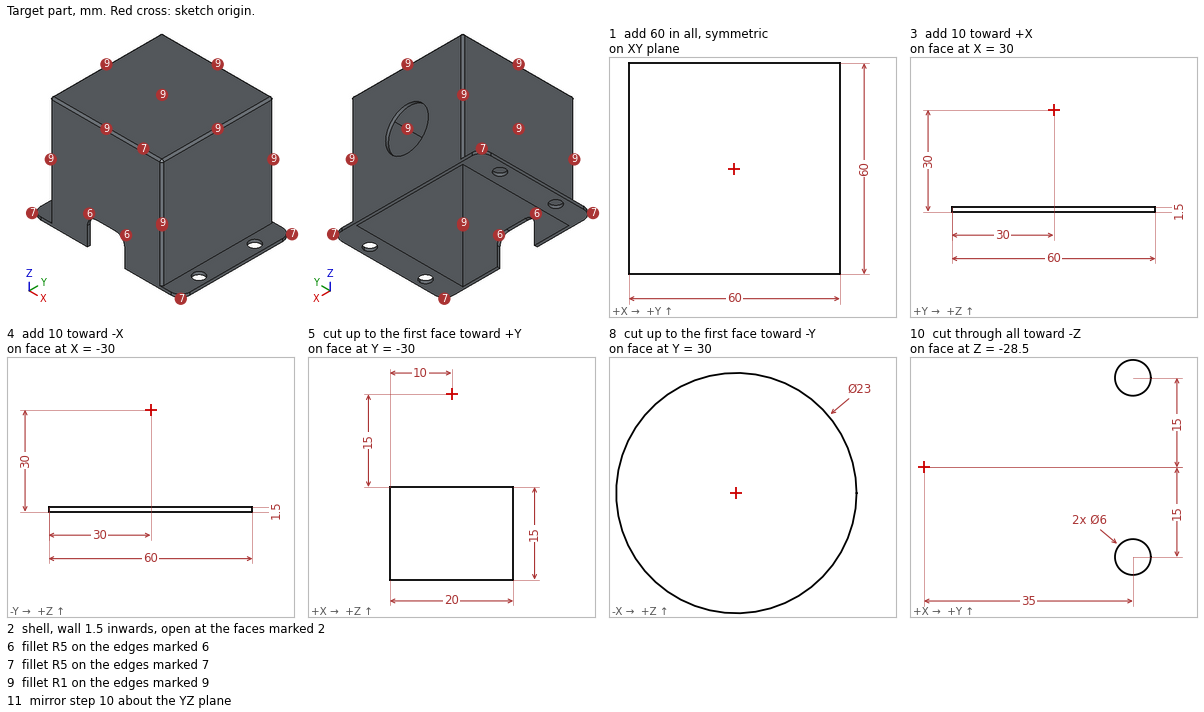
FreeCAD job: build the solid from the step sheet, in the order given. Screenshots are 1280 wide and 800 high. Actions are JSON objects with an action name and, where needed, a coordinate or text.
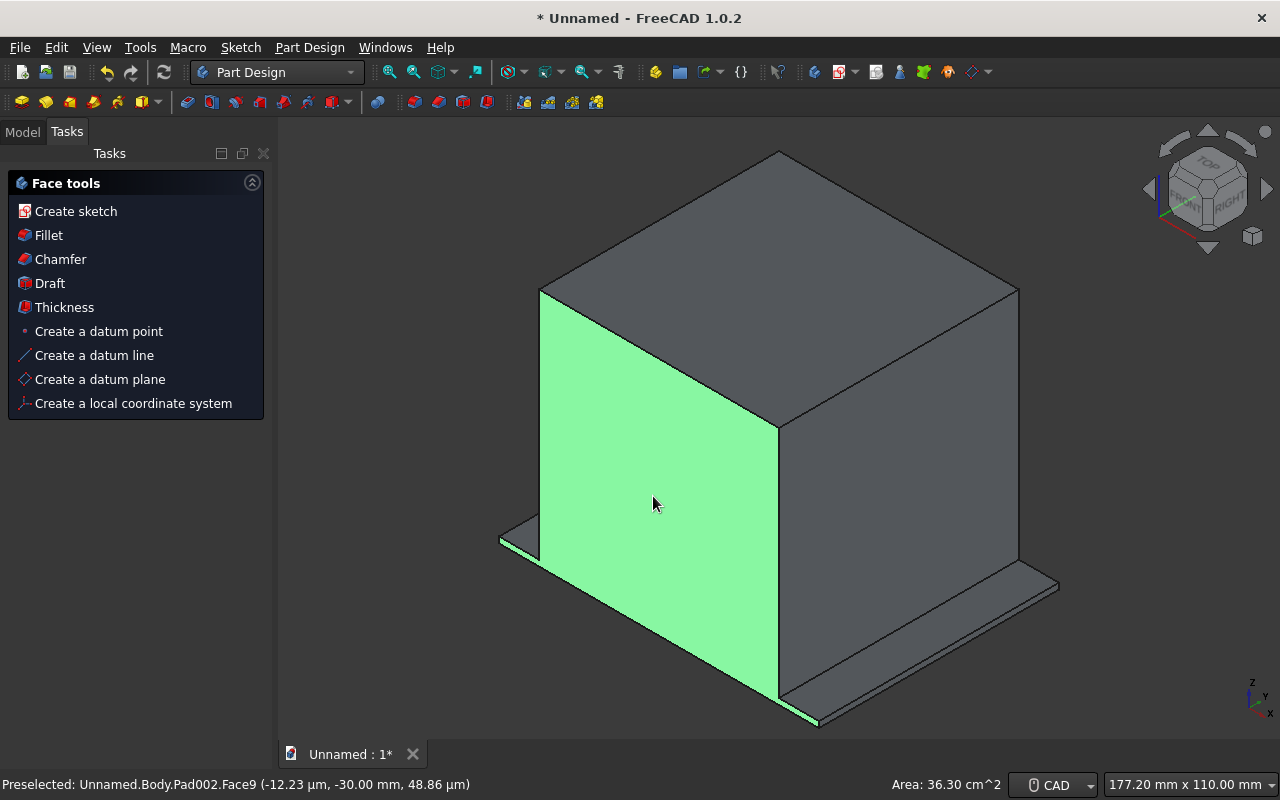
{"action": "left_click", "coordinate": [840, 72]}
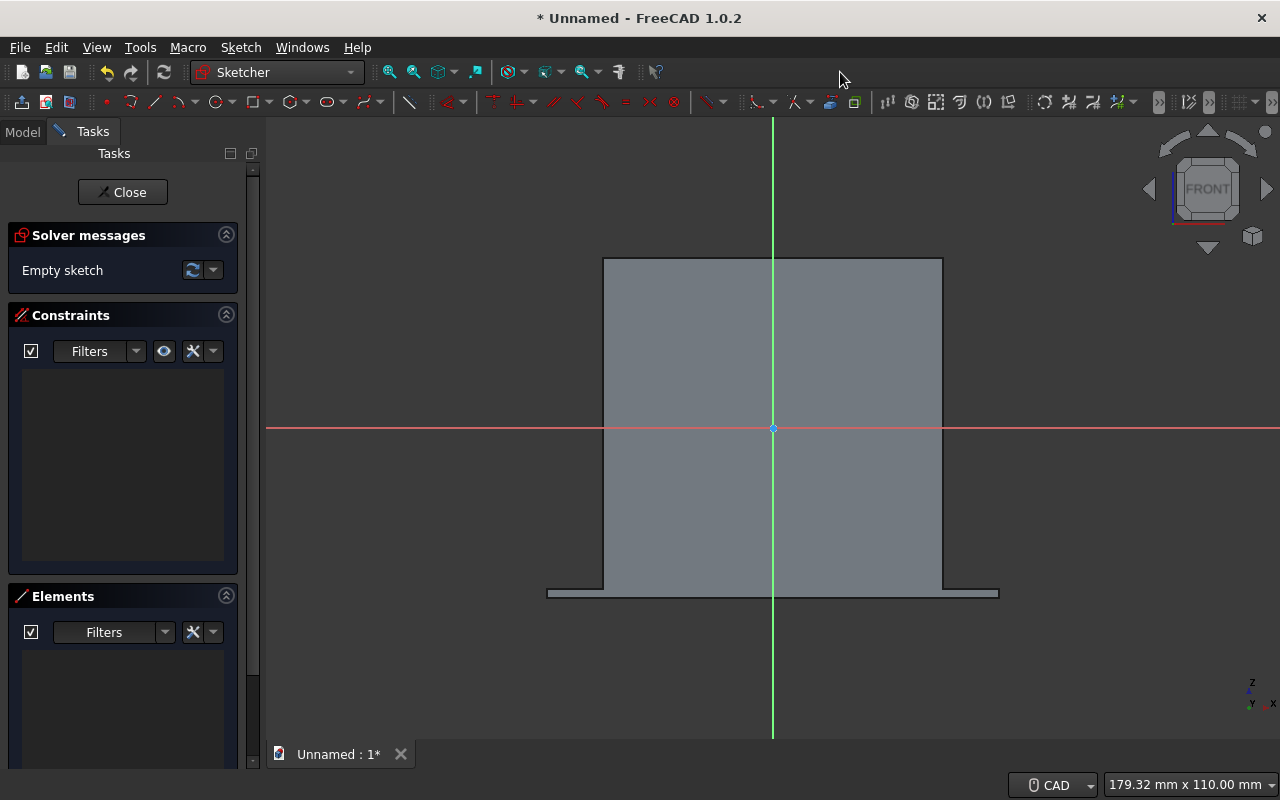
{"action": "scroll", "coordinate": [829, 582], "scroll_direction": "up", "scroll_amount": 4}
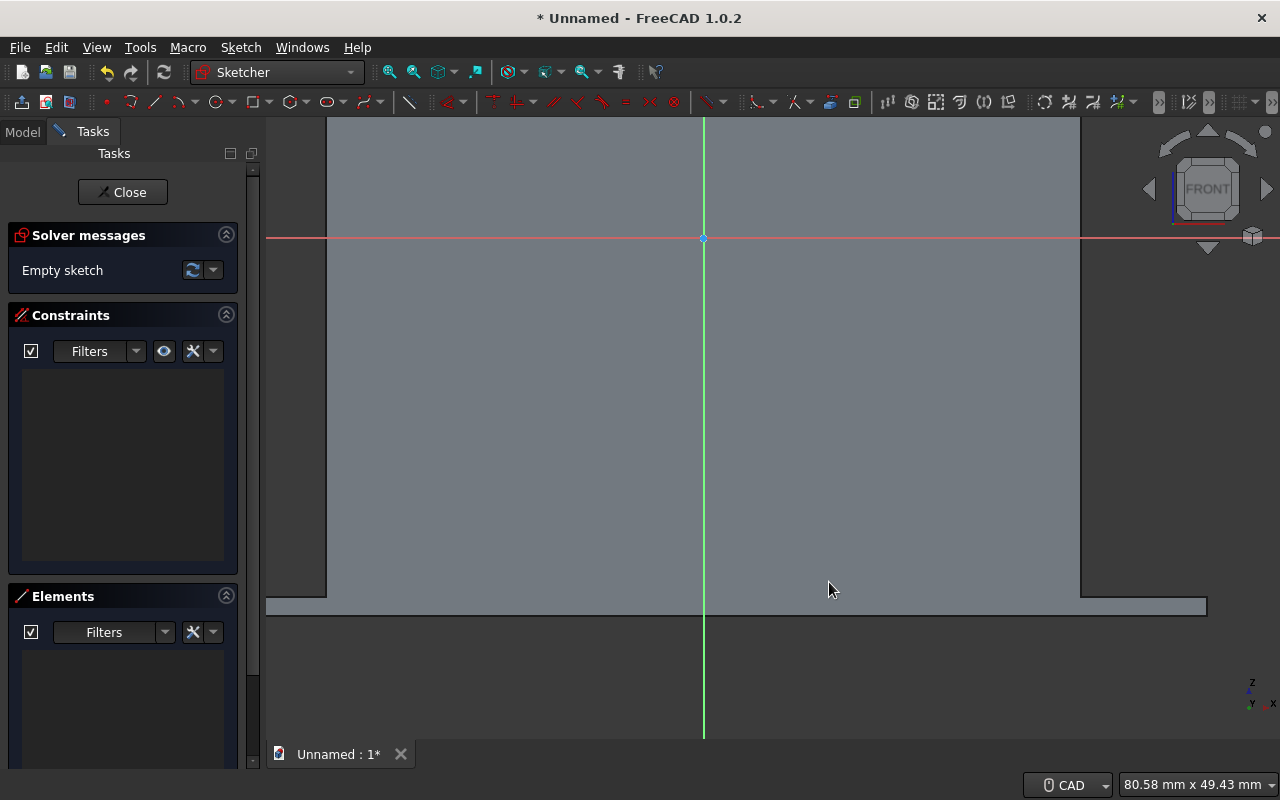
{"action": "left_click", "coordinate": [254, 102]}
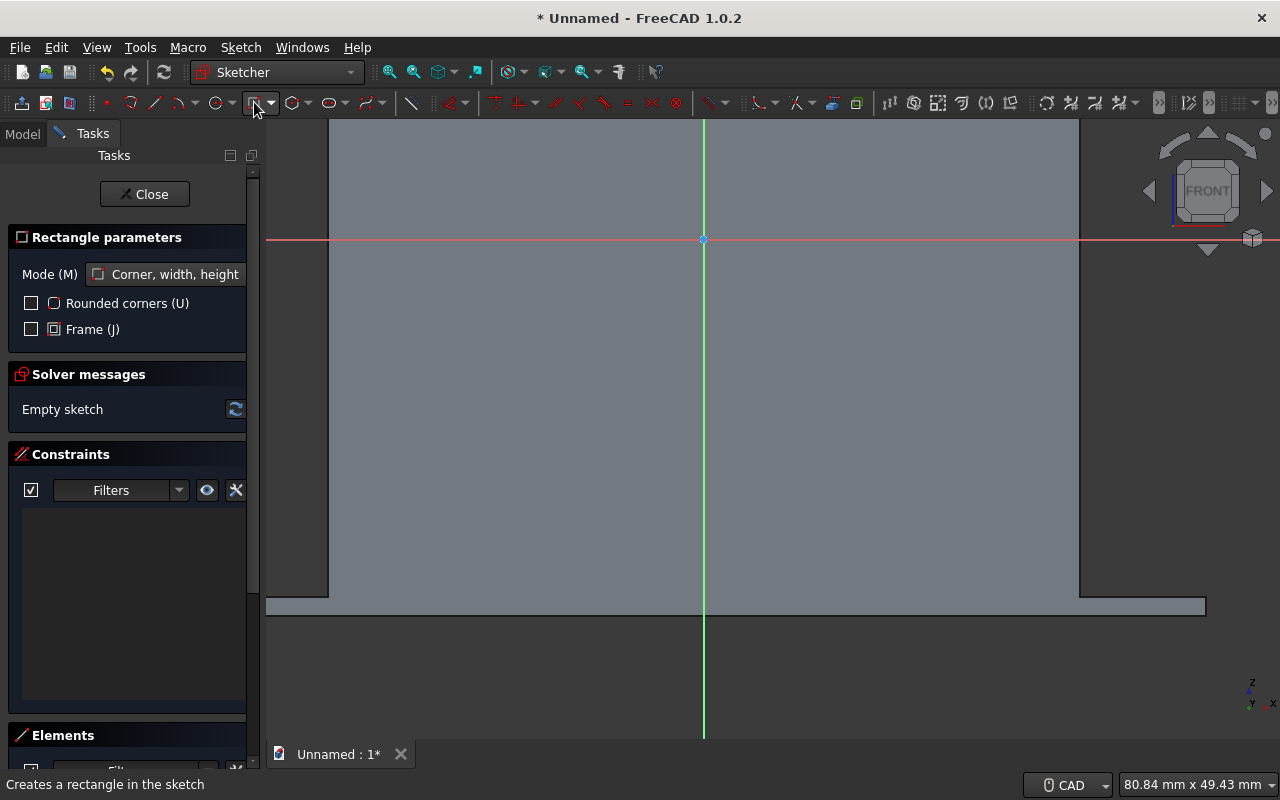
{"action": "left_click", "coordinate": [578, 428]}
{"action": "mouse_move", "coordinate": [829, 616]}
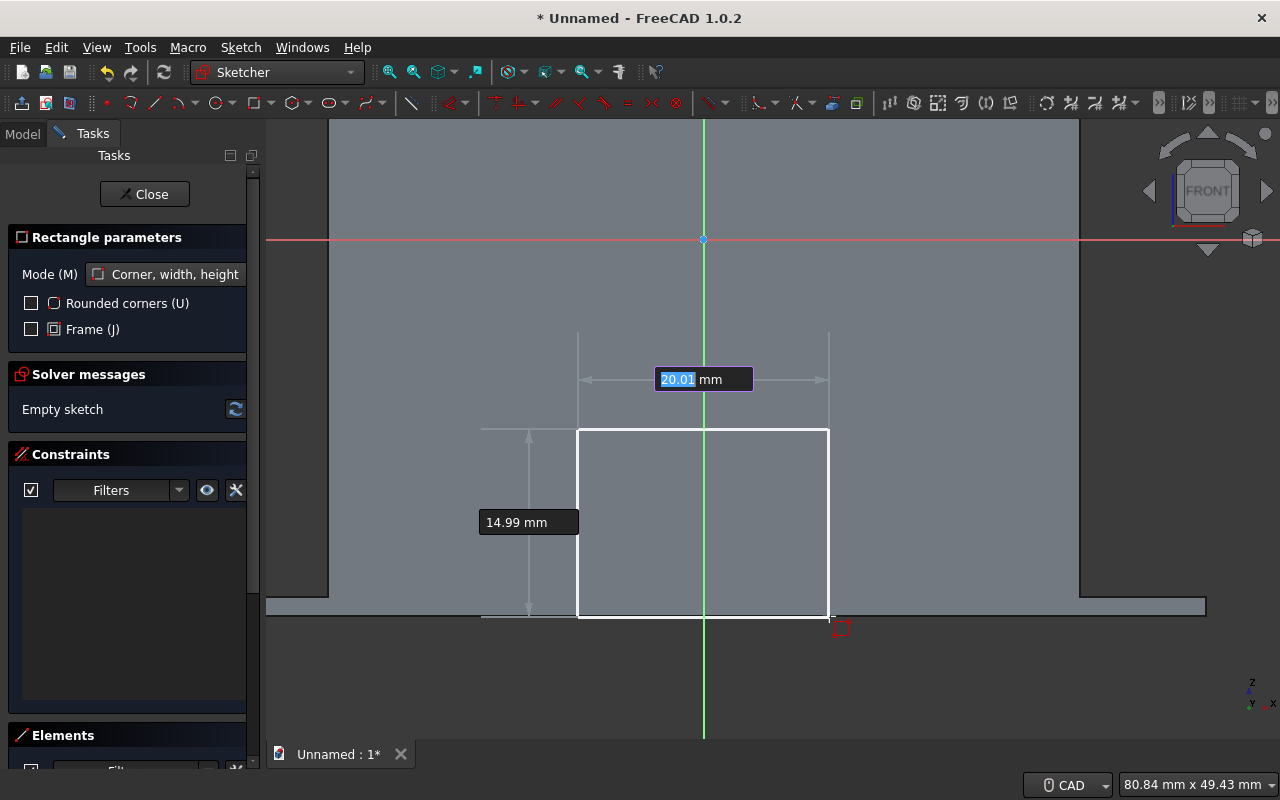
{"action": "type", "text": "20"}
{"action": "key", "text": "Tab"}
{"action": "type", "text": "15"}
{"action": "key", "text": "Return"}
{"action": "key", "text": "Escape"}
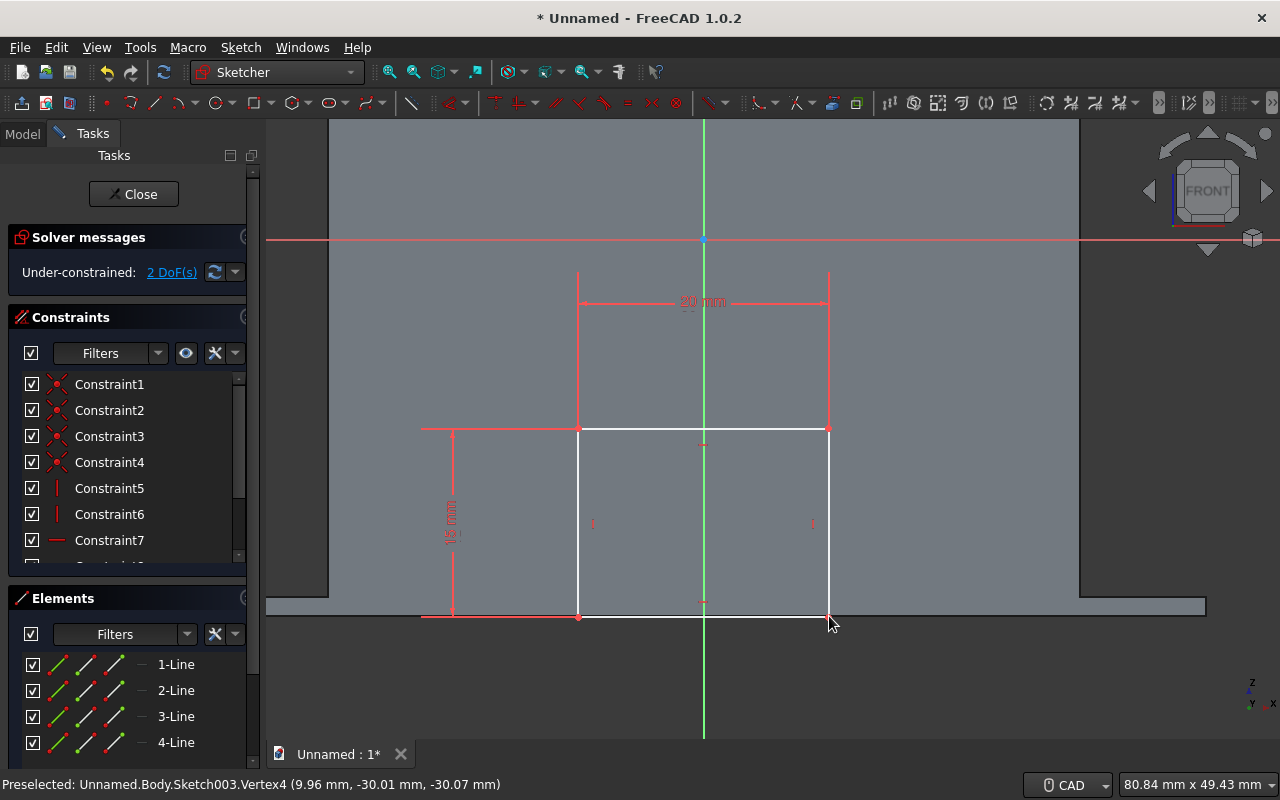
{"action": "left_click", "coordinate": [578, 429]}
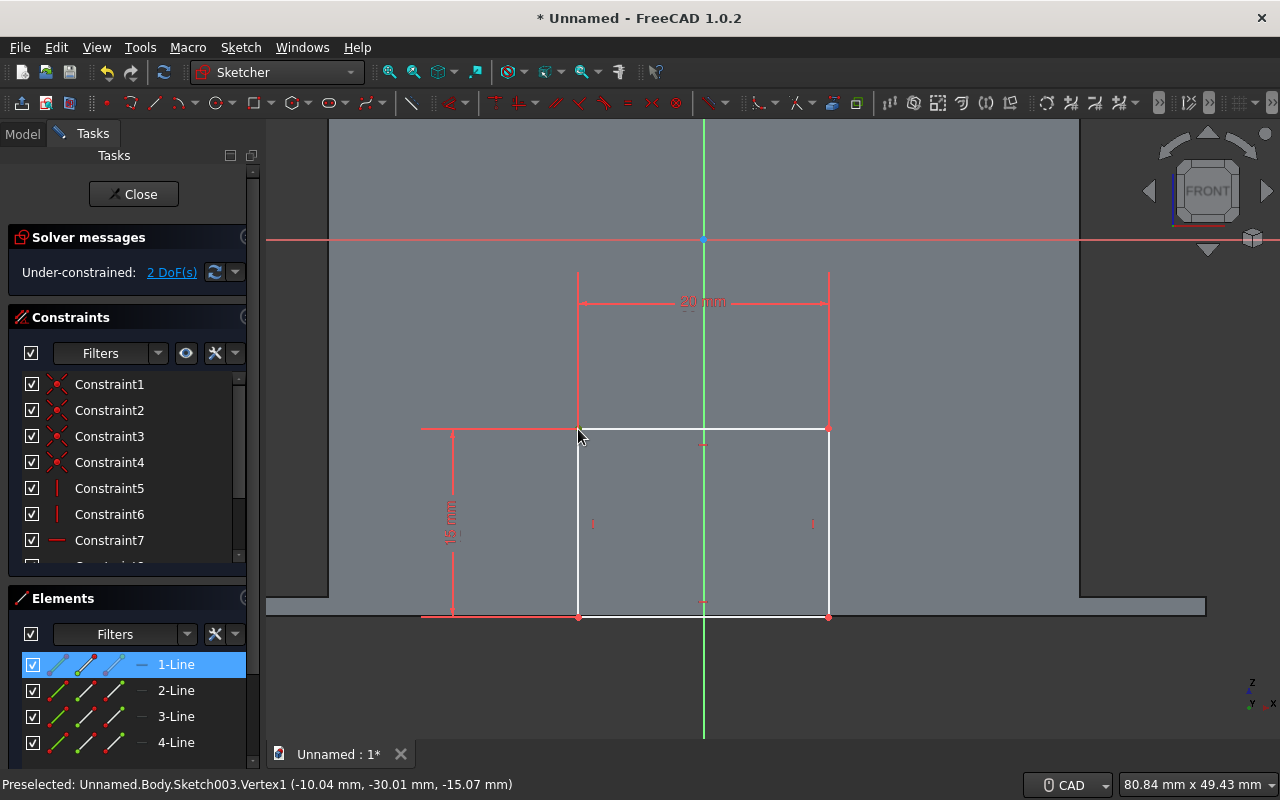
{"action": "left_click", "coordinate": [468, 104]}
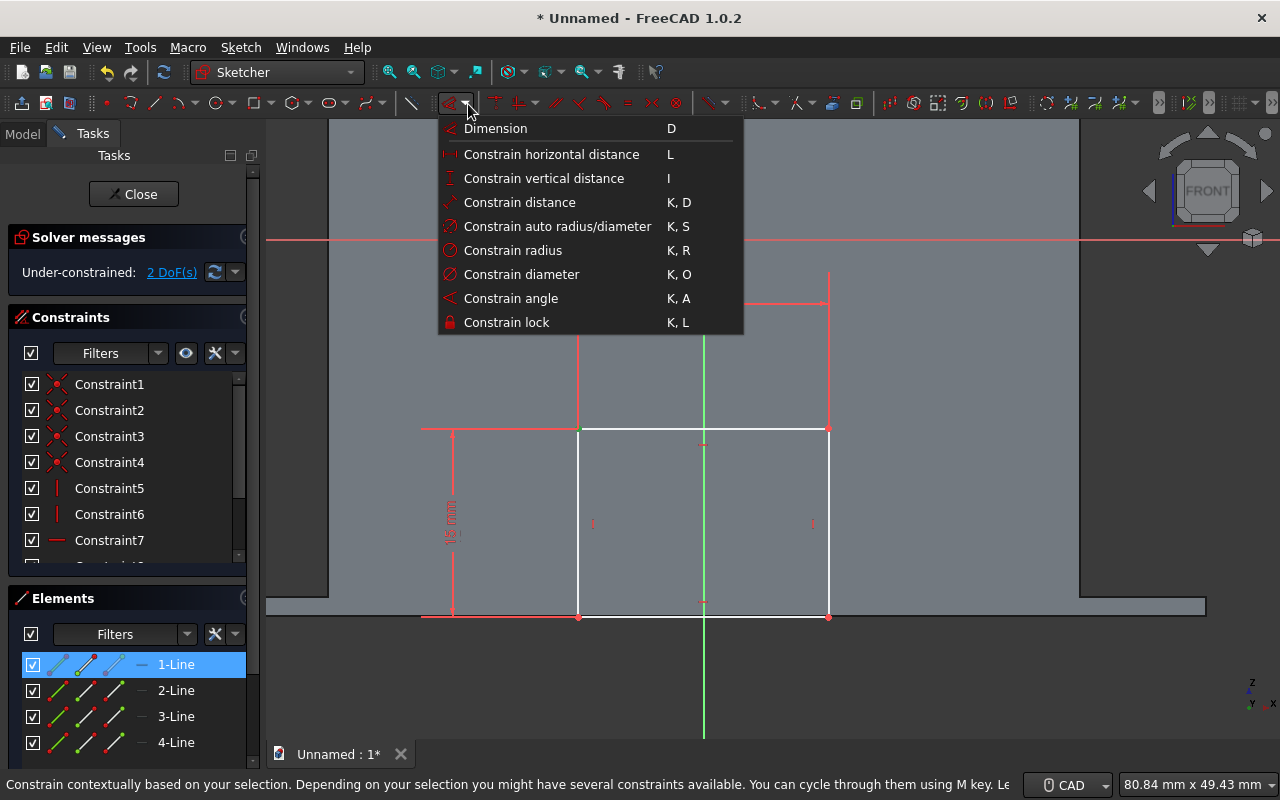
{"action": "left_click", "coordinate": [591, 154]}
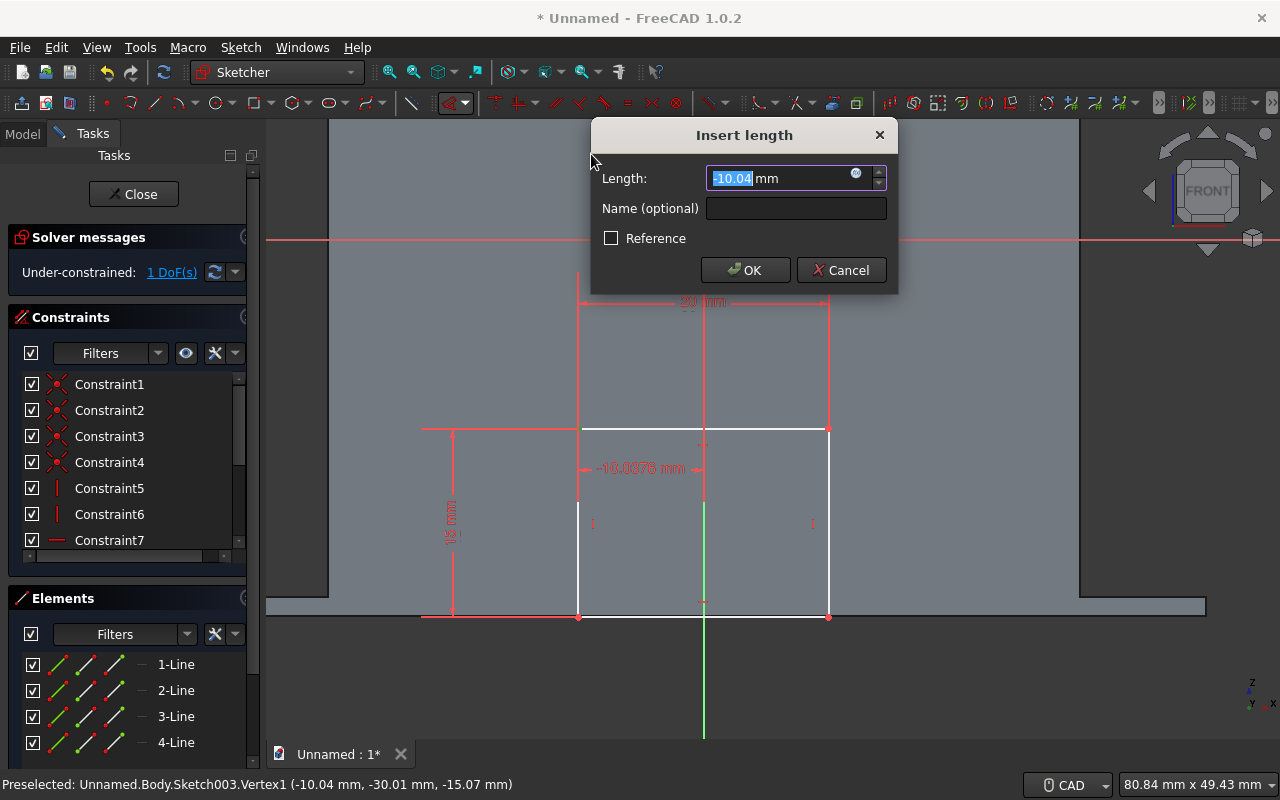
{"action": "type", "text": "-10"}
{"action": "key", "text": "Return"}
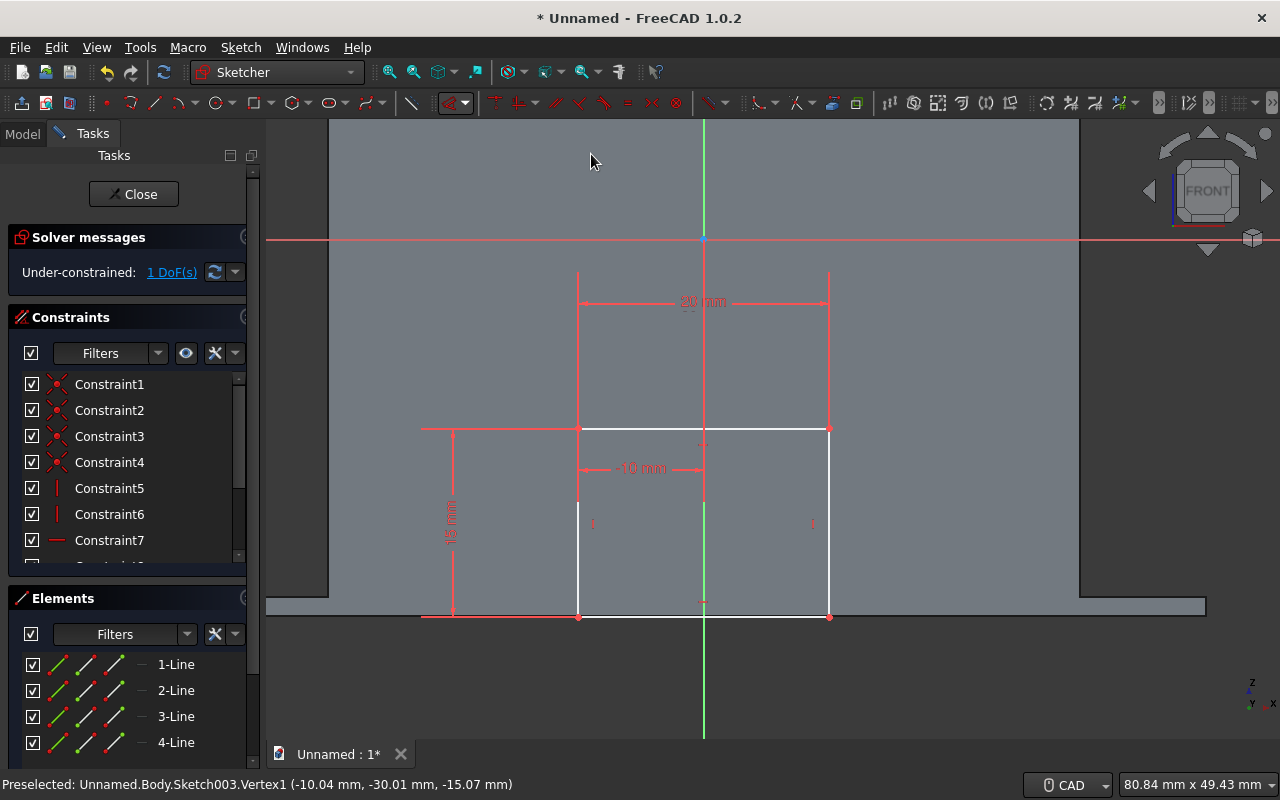
{"action": "left_click", "coordinate": [578, 429]}